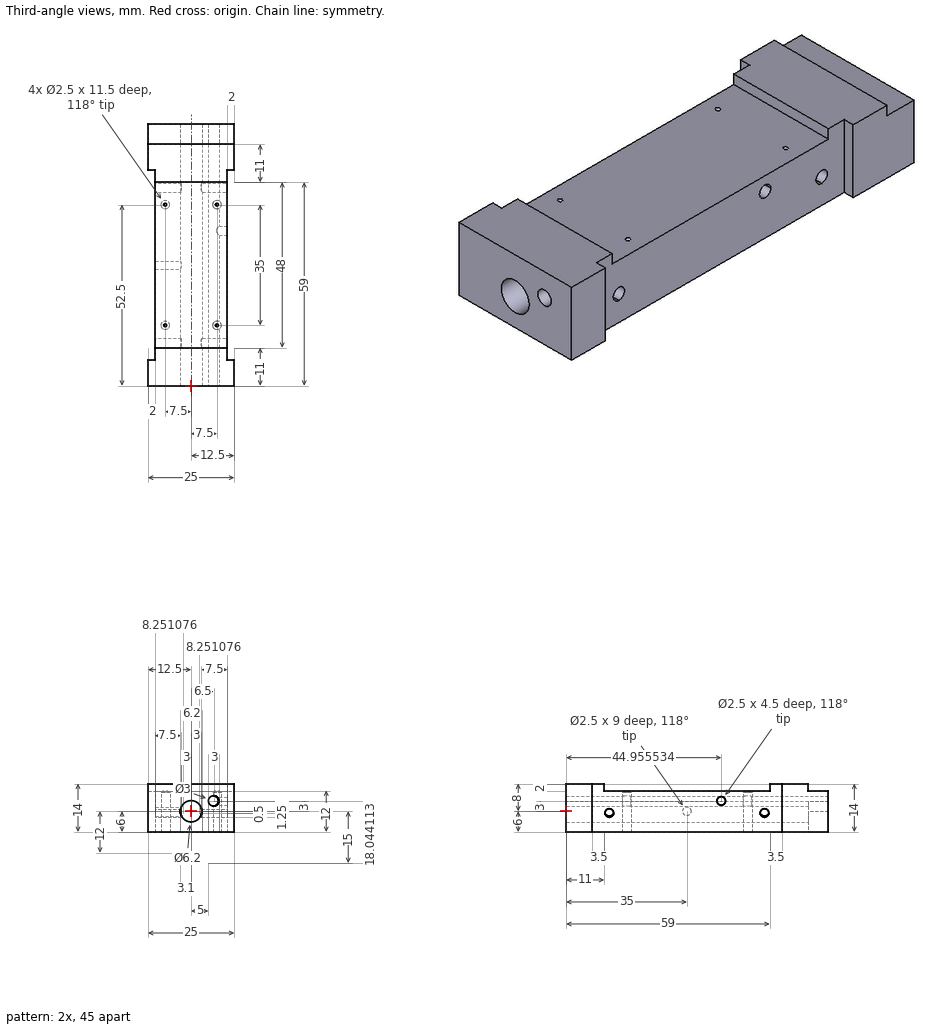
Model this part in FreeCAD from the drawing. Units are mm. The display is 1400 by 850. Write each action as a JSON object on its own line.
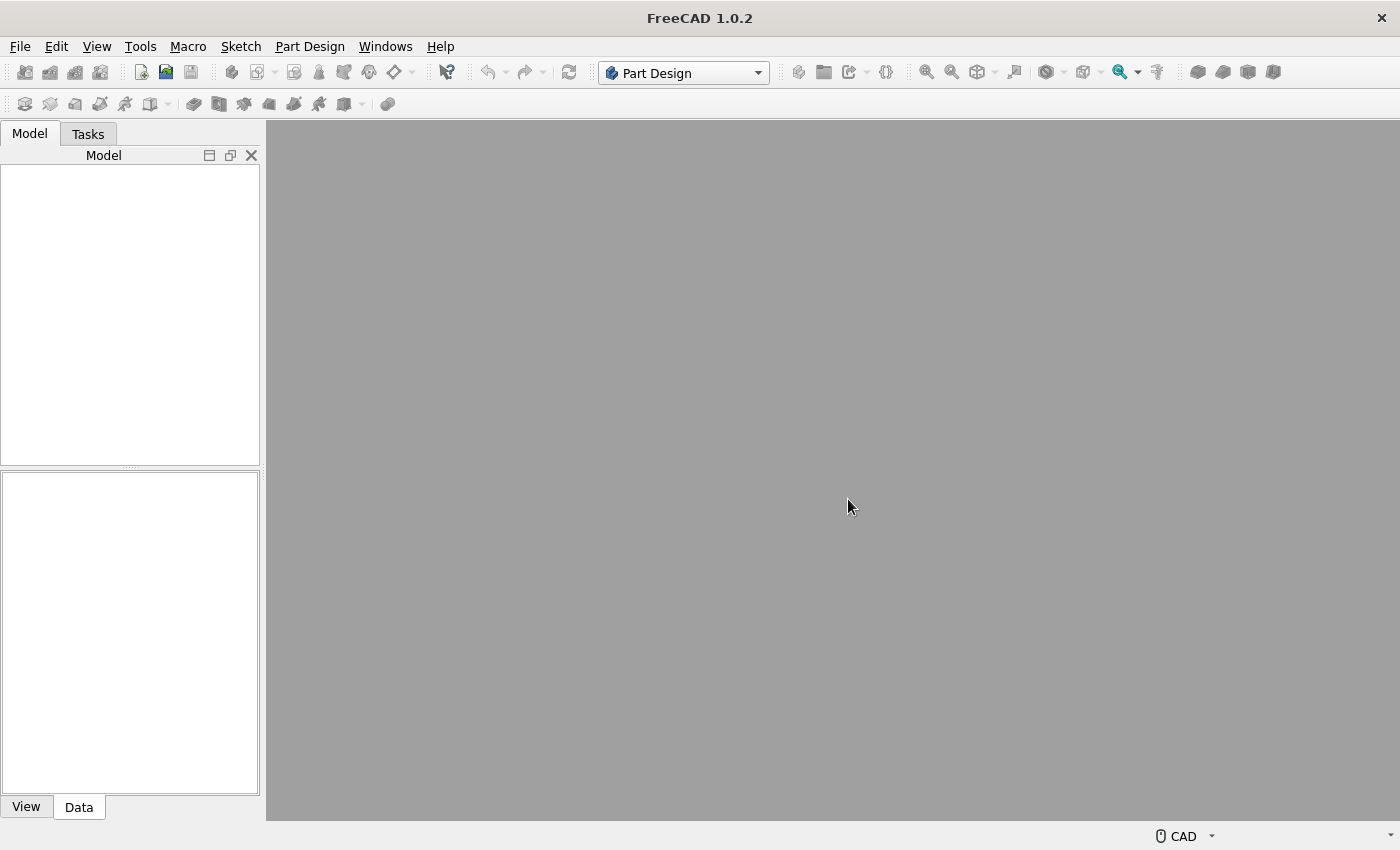
{"action": "left_click", "coordinate": [141, 72]}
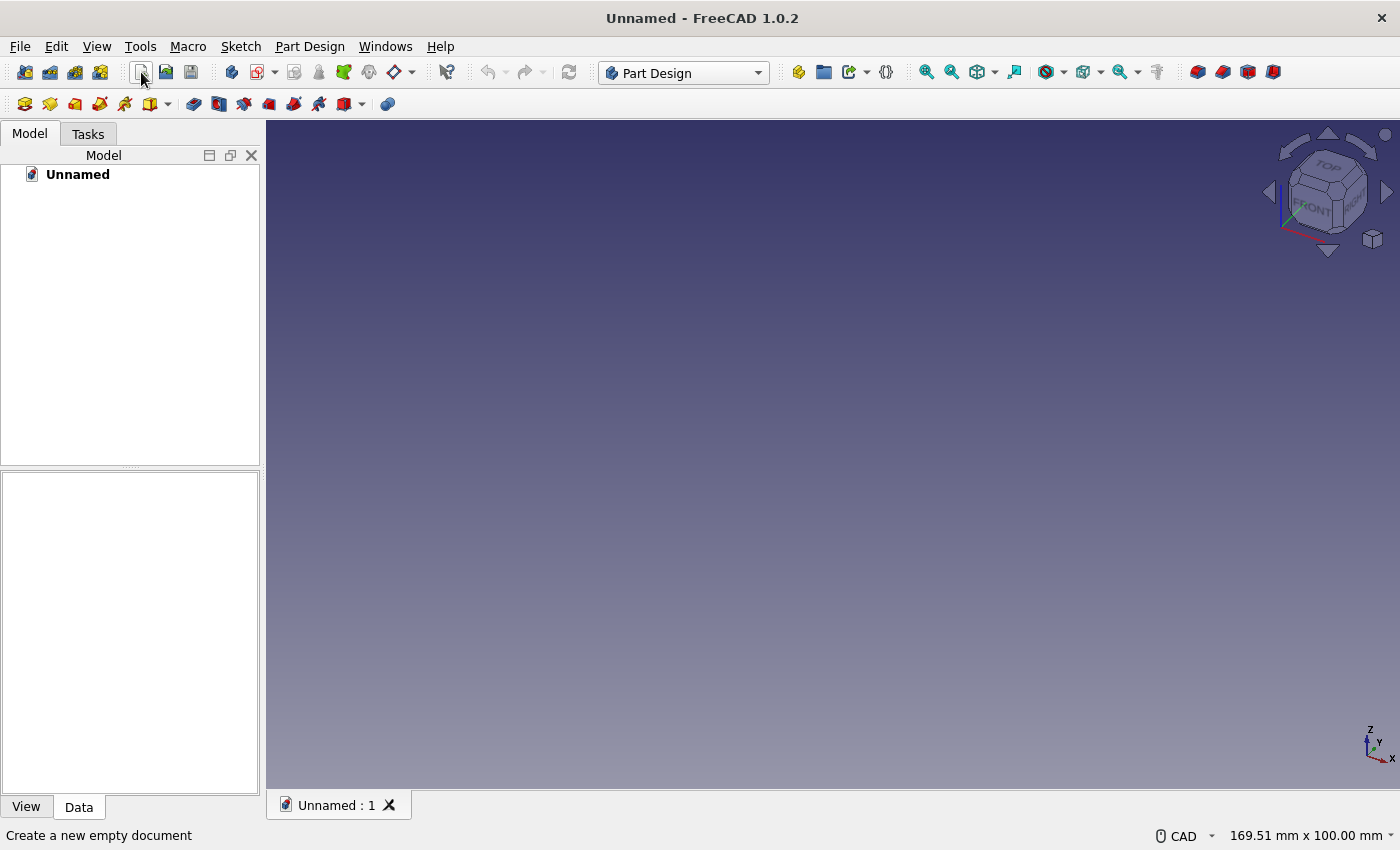
{"action": "left_click", "coordinate": [256, 72]}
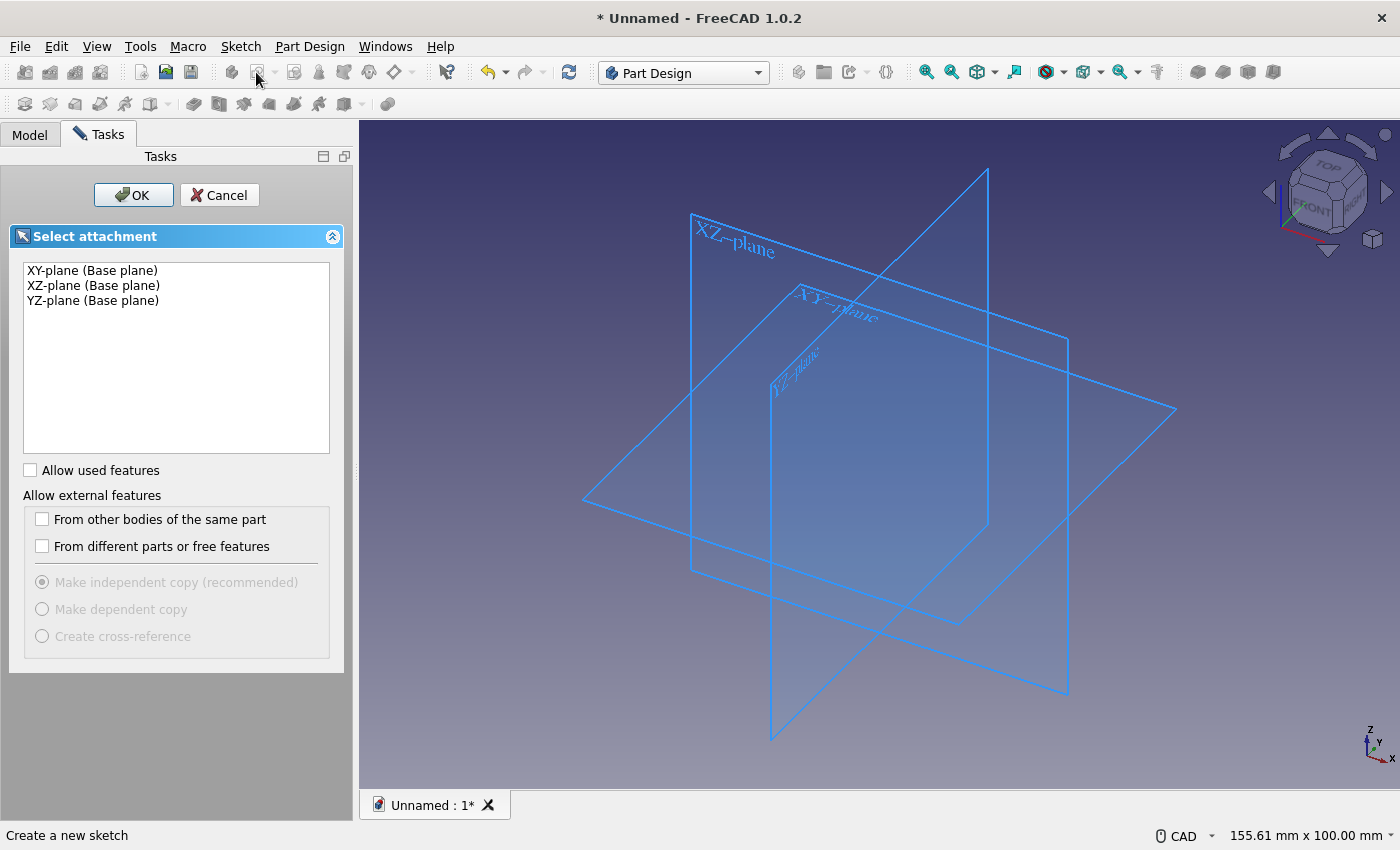
{"action": "left_click", "coordinate": [84, 286]}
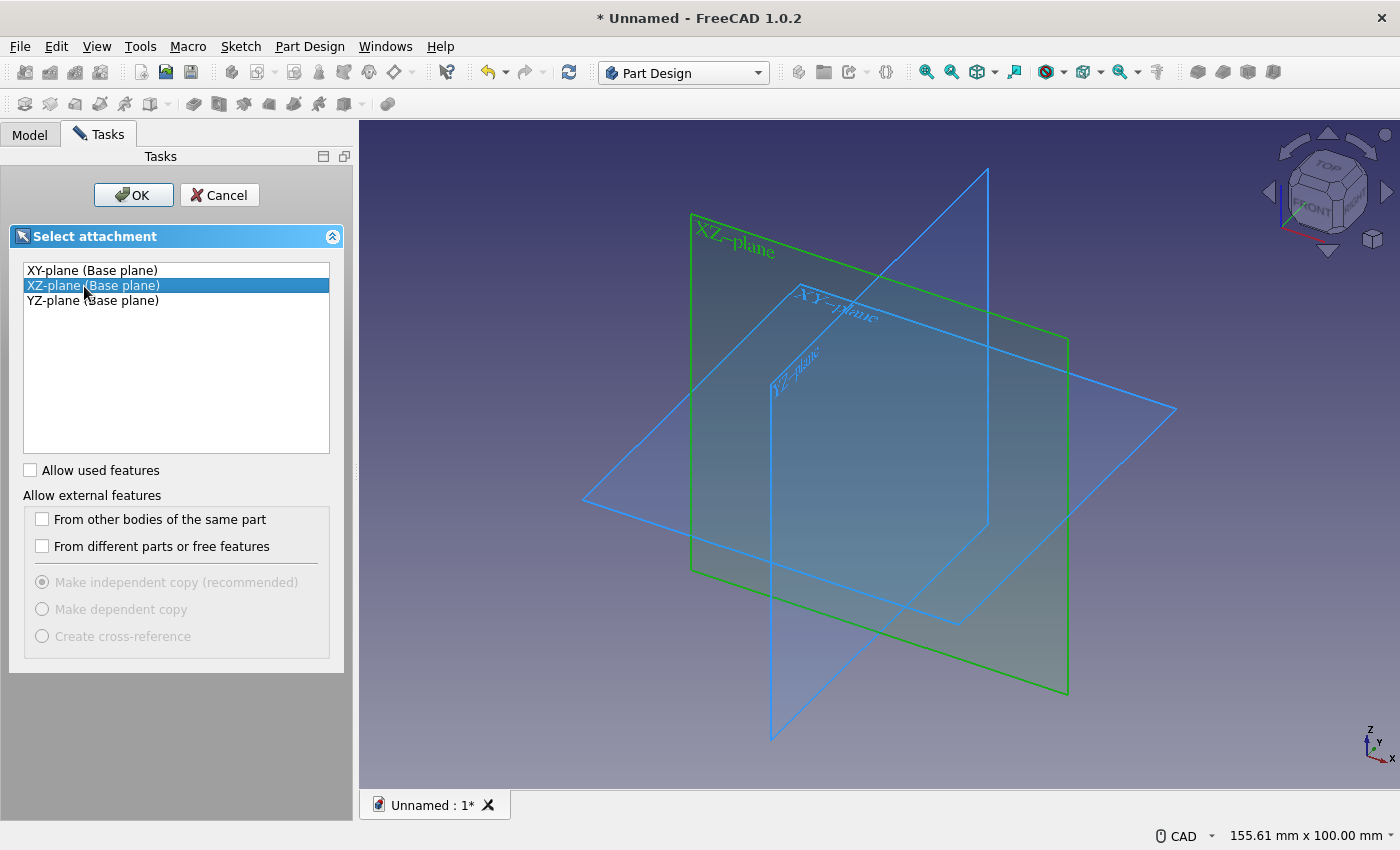
{"action": "left_click", "coordinate": [134, 195]}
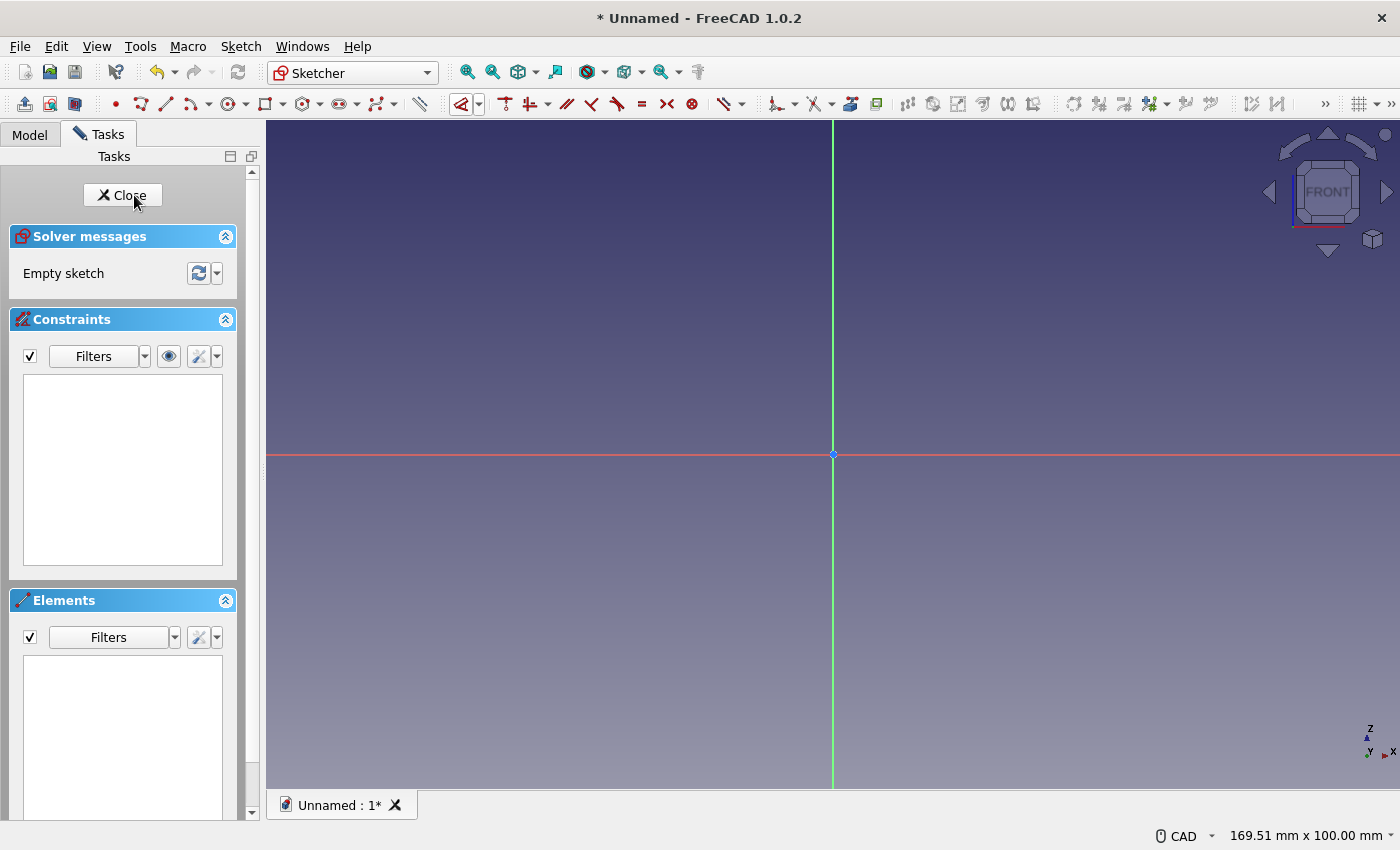
{"action": "scroll", "coordinate": [855, 454], "scroll_direction": "up", "scroll_amount": 7}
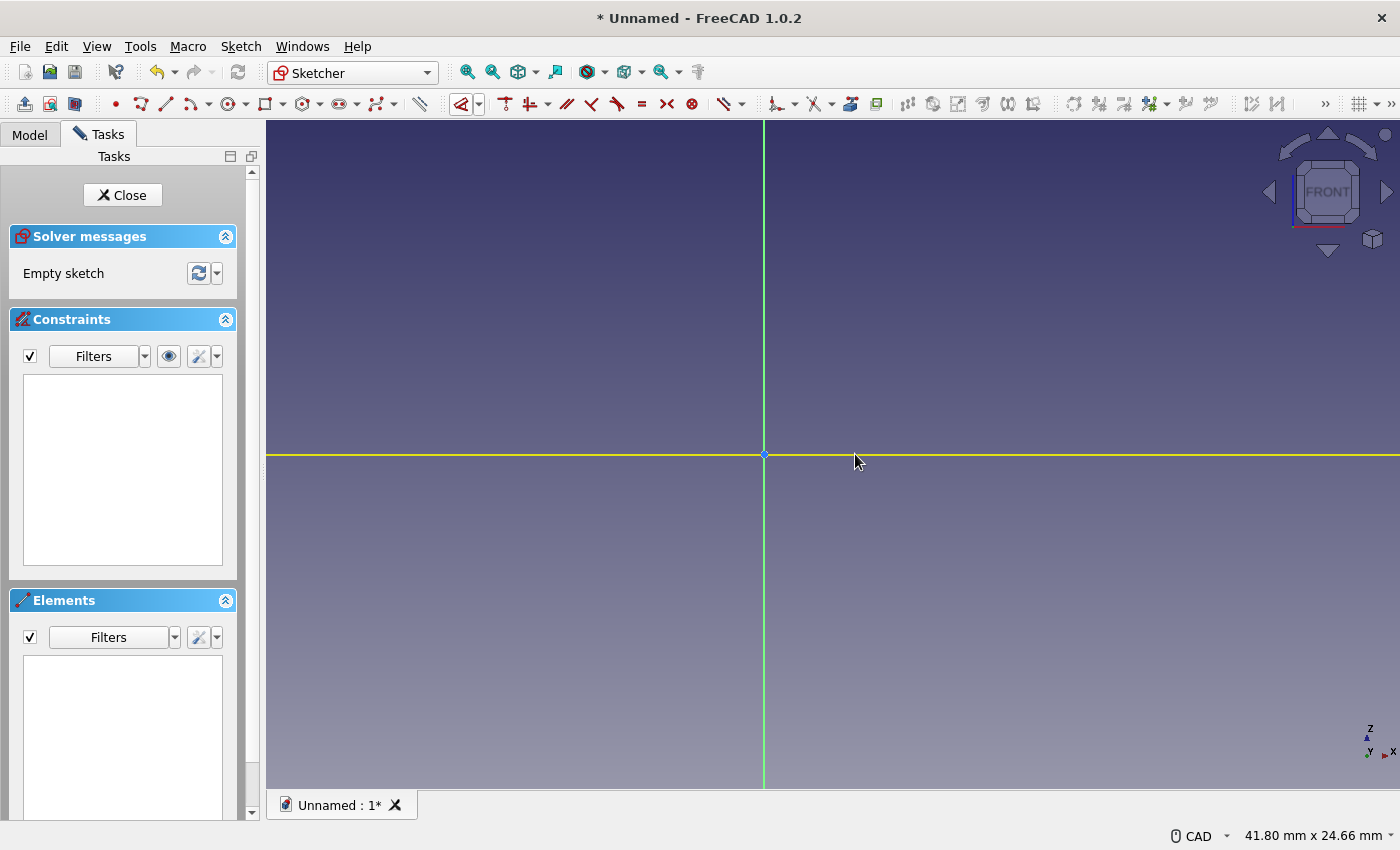
{"action": "left_click", "coordinate": [282, 104]}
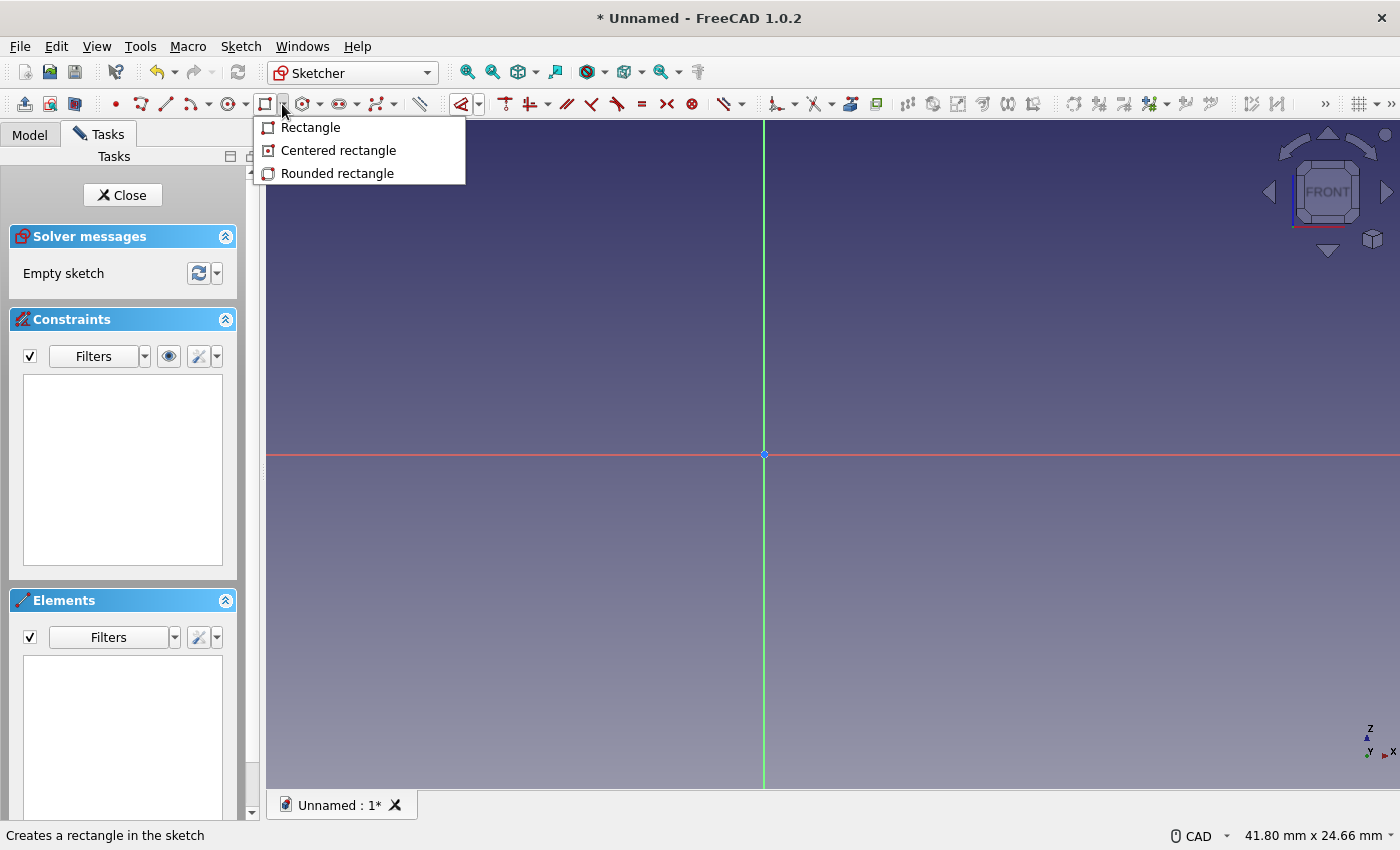
{"action": "left_click", "coordinate": [360, 150]}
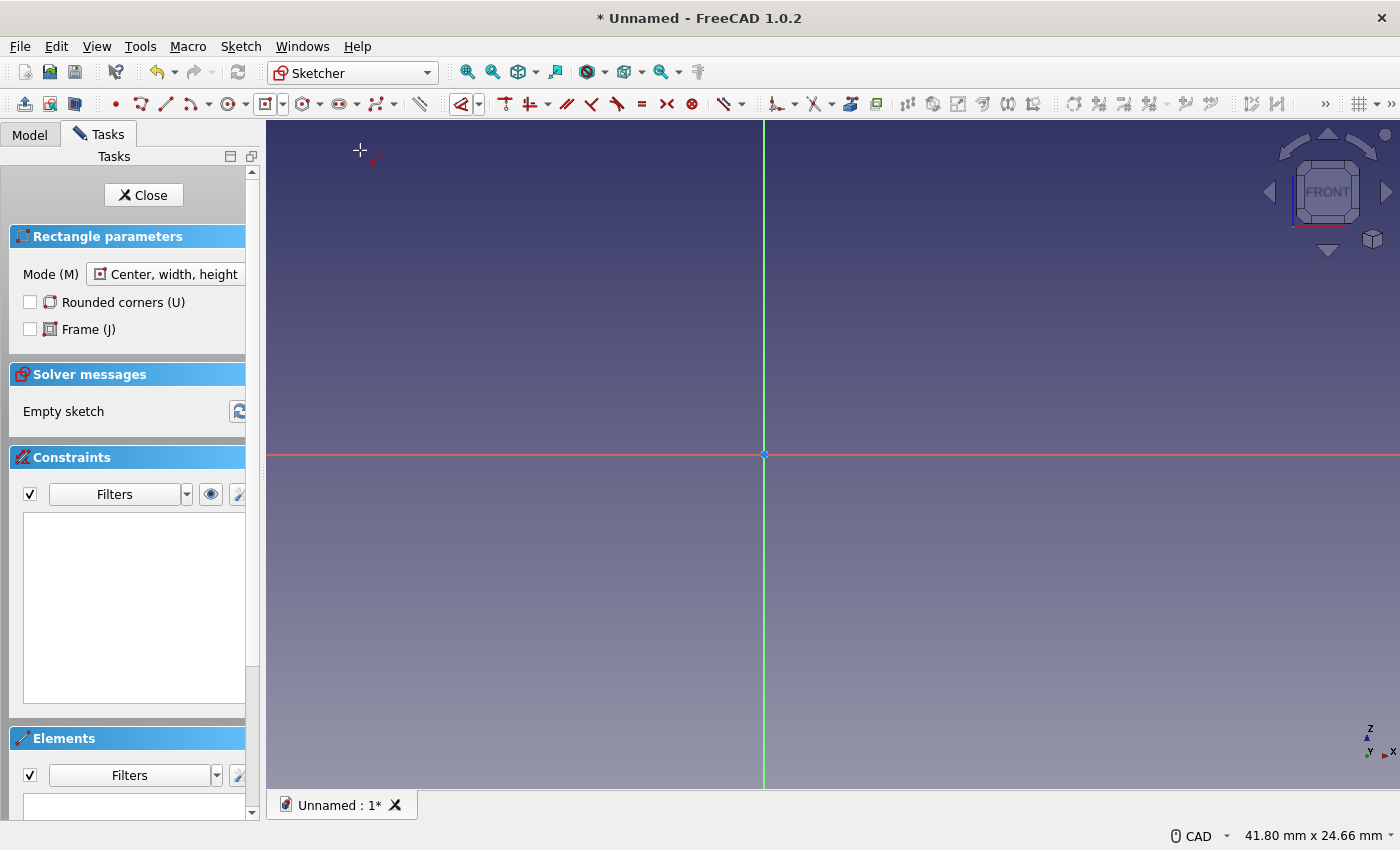
{"action": "left_click", "coordinate": [764, 454]}
{"action": "left_click", "coordinate": [1103, 292]}
{"action": "key", "text": "Escape"}